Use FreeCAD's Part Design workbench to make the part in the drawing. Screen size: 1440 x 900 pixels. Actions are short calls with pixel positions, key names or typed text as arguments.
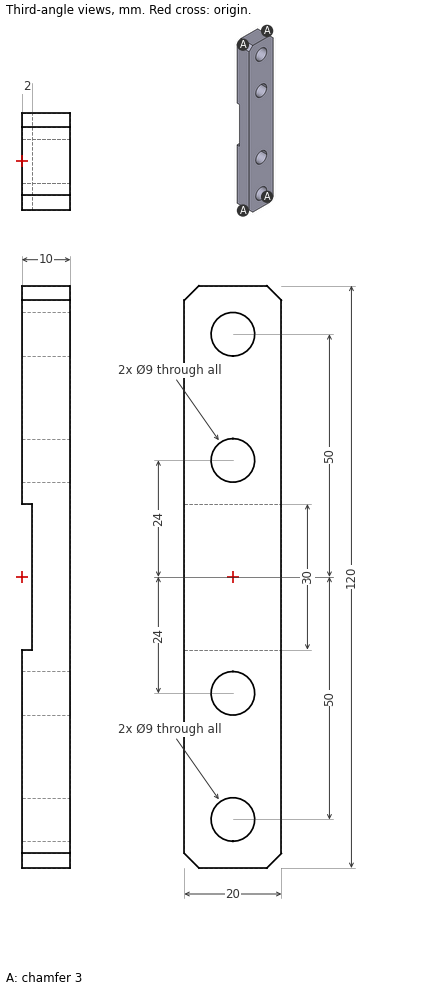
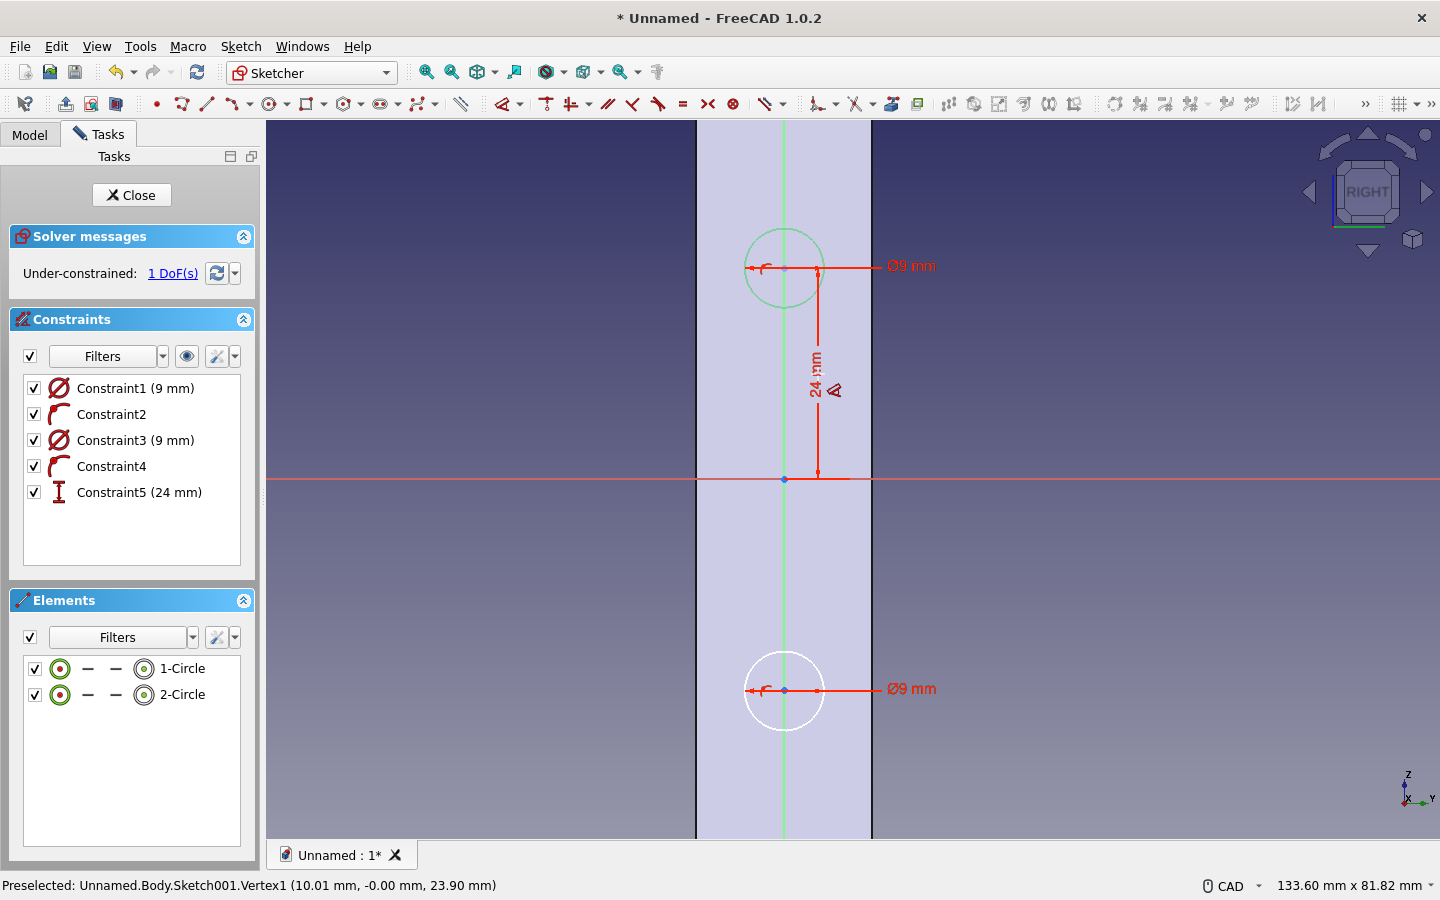
click(784, 691)
click(818, 585)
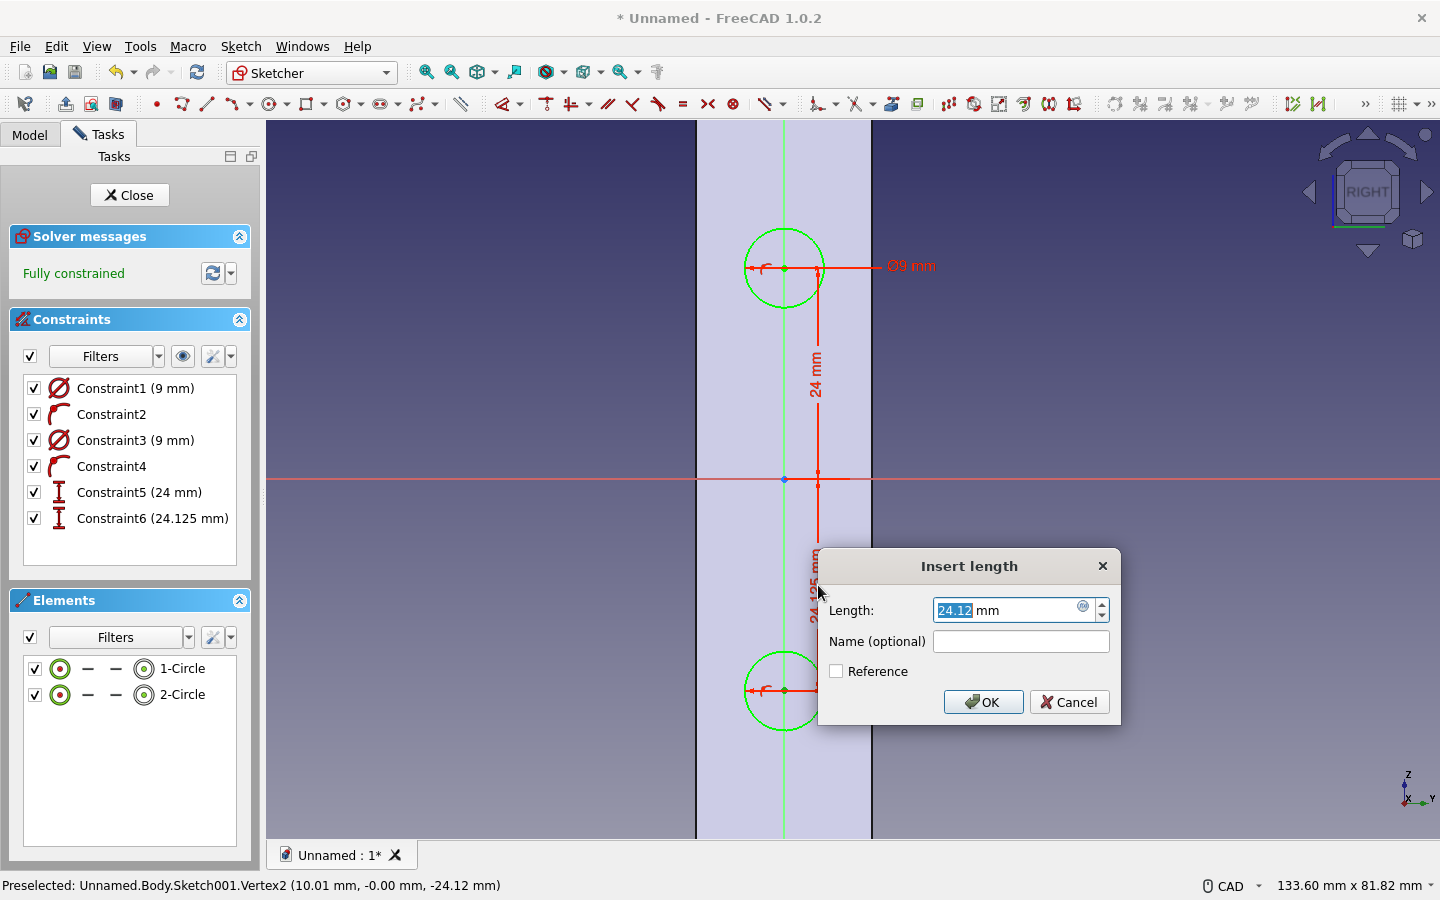
text(24)
key(Return)
key(Escape)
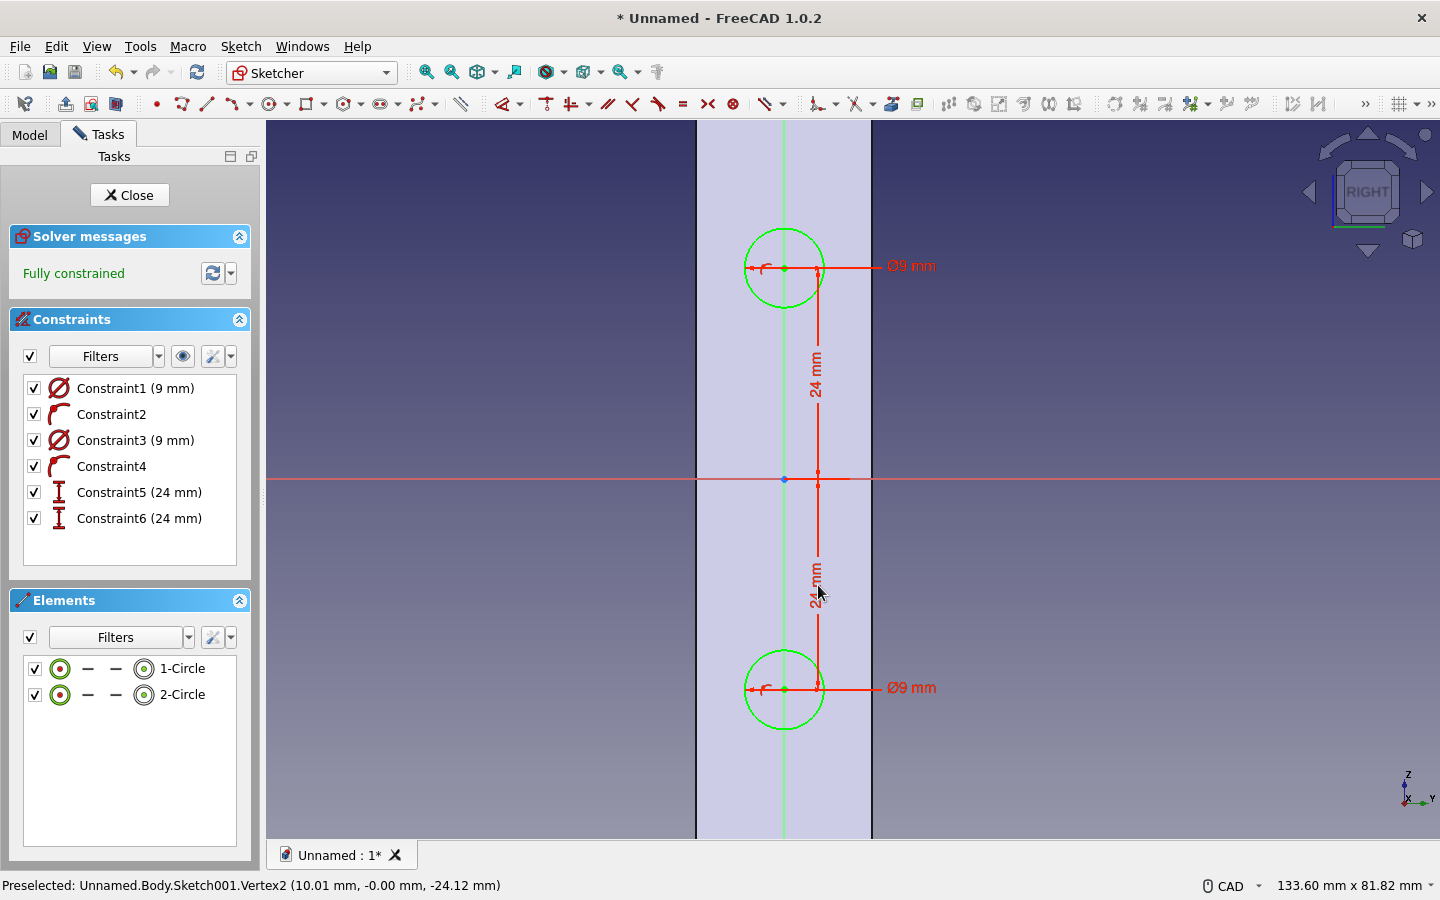
click(130, 195)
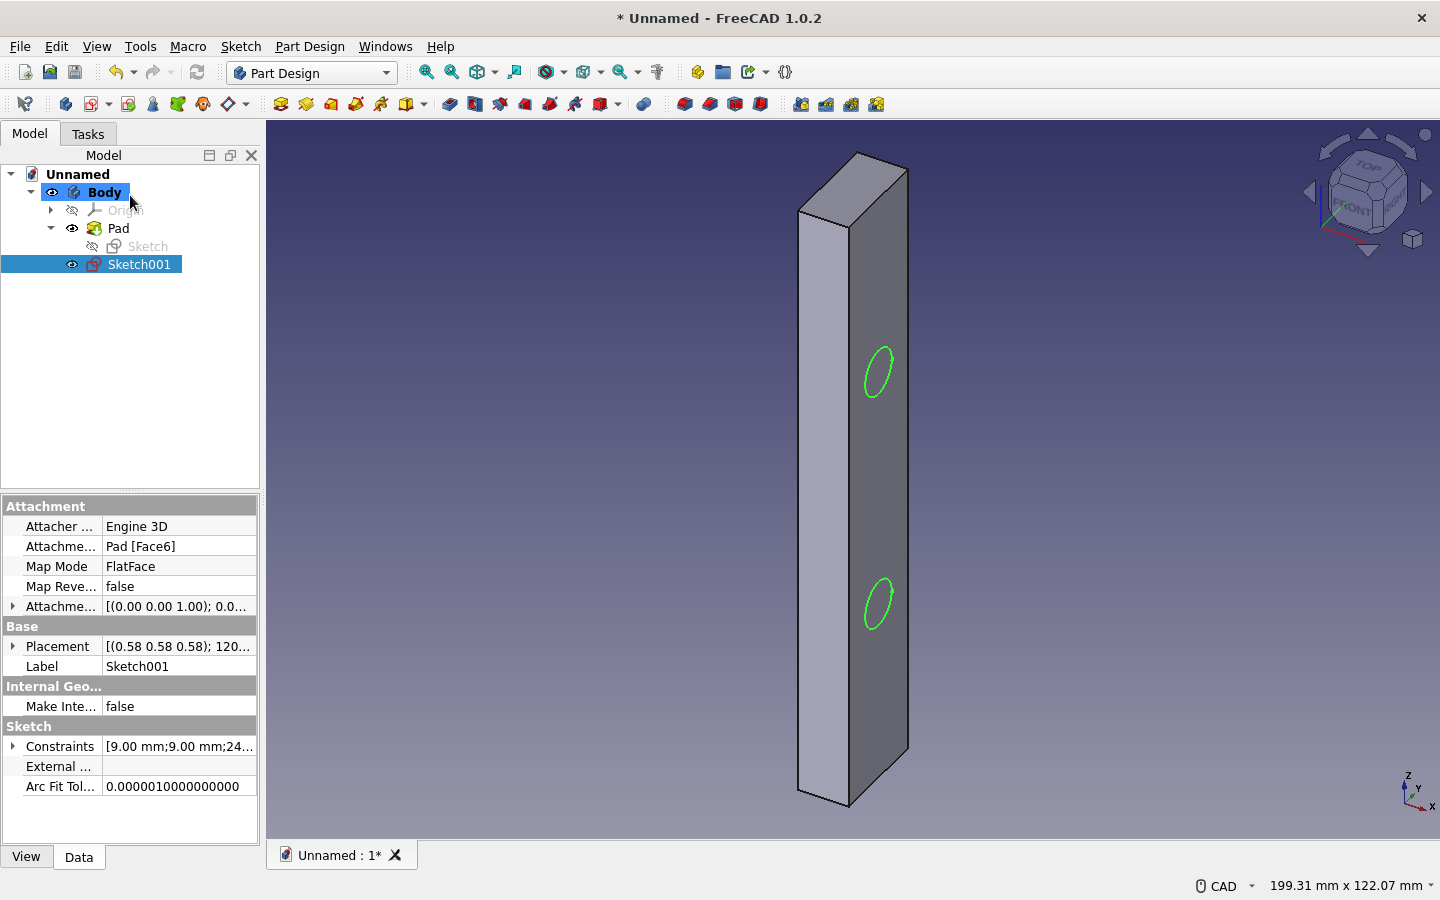
click(475, 104)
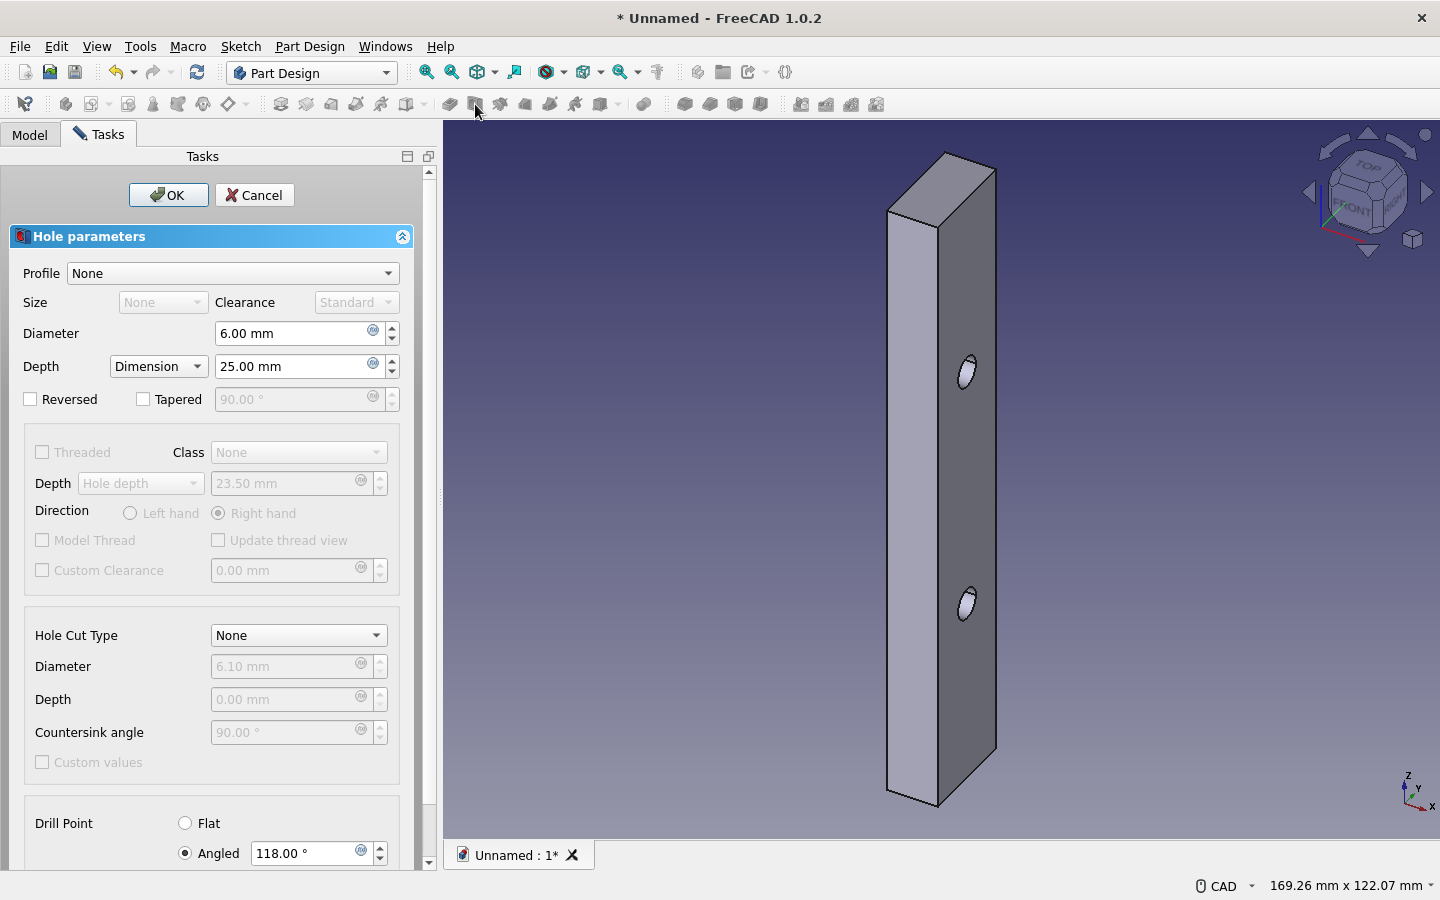
triple_click(300, 334)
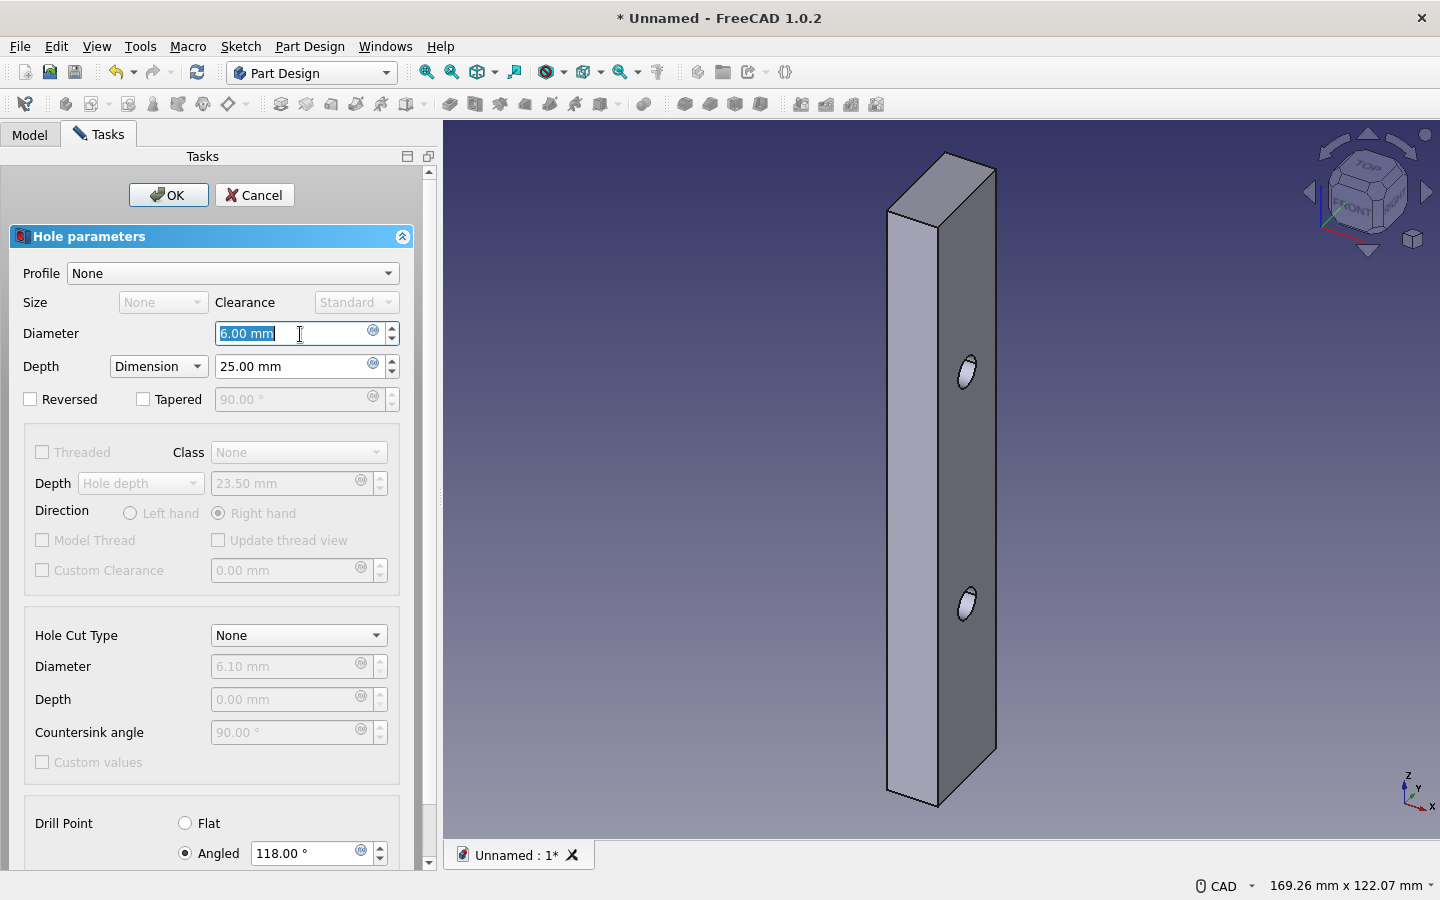
text(9)
key(Tab)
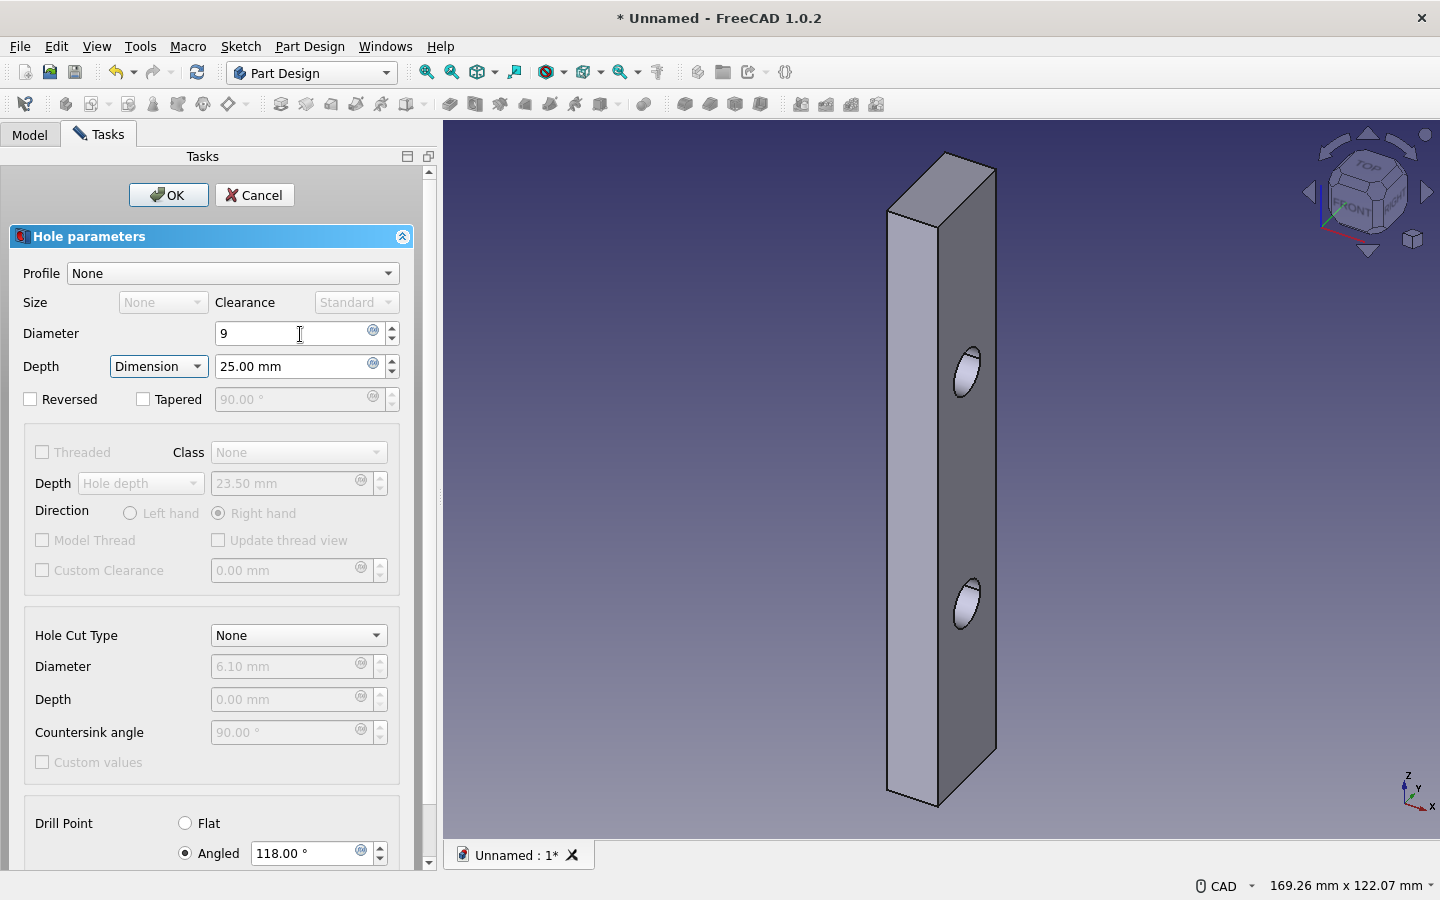
click(160, 366)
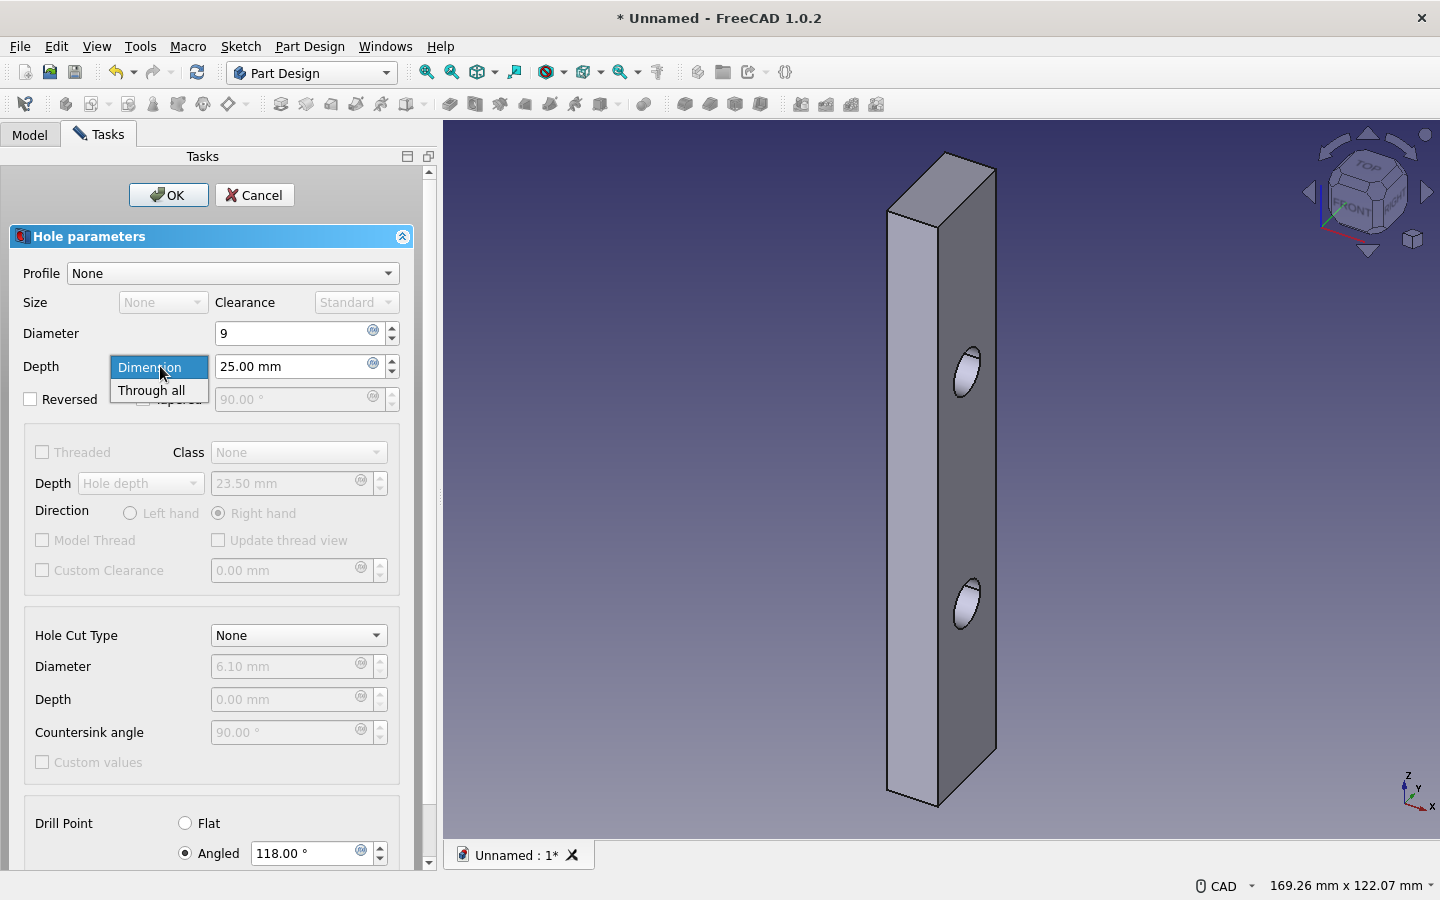
click(158, 390)